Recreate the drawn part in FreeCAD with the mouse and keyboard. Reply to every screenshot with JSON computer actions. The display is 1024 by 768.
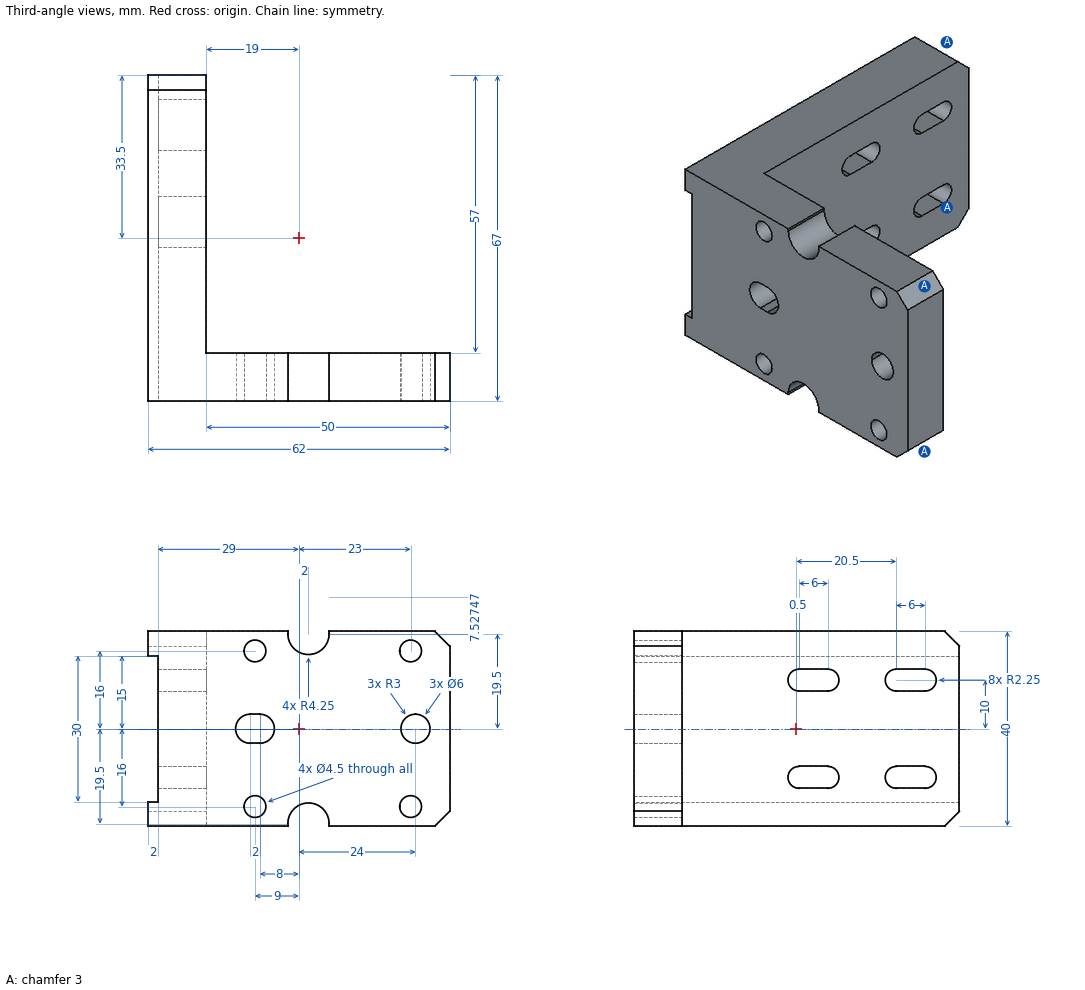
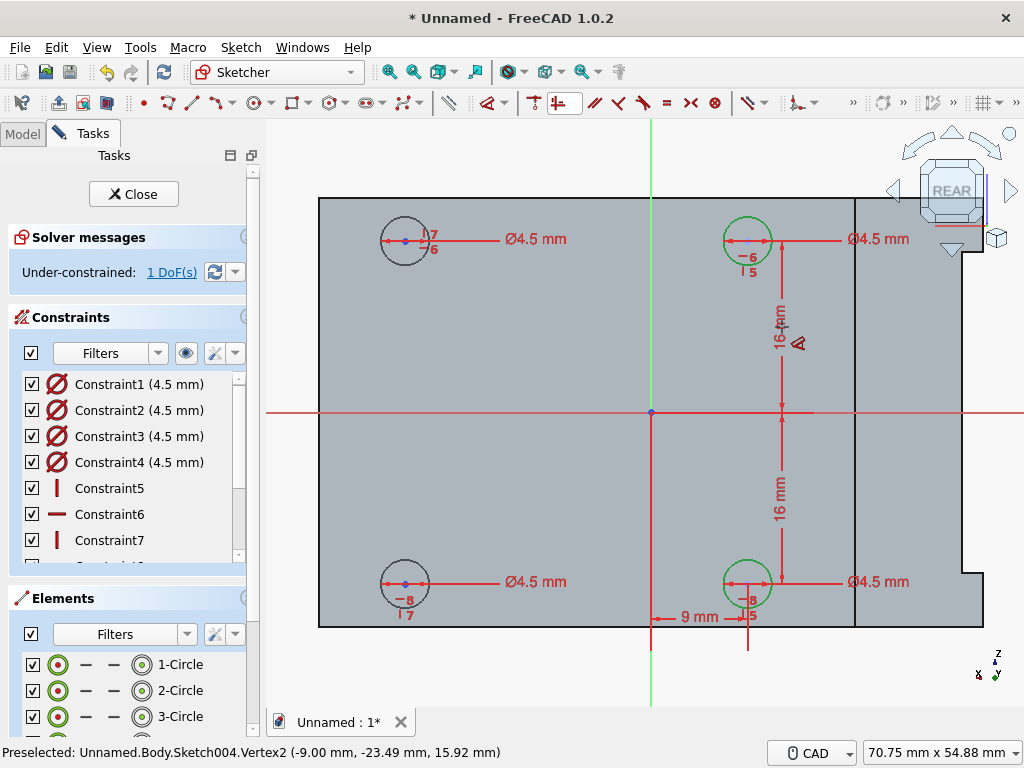
{"action": "left_click", "coordinate": [405, 241]}
{"action": "left_click", "coordinate": [528, 207]}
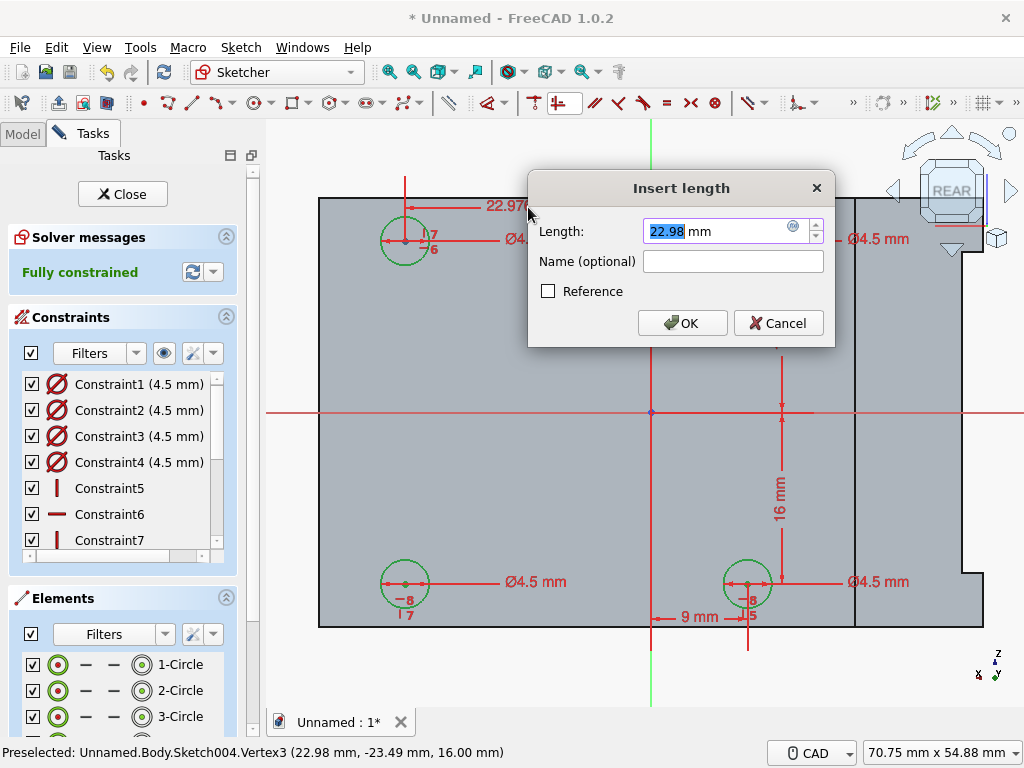
{"action": "type", "text": "23"}
{"action": "key", "text": "Return"}
{"action": "key", "text": "Escape"}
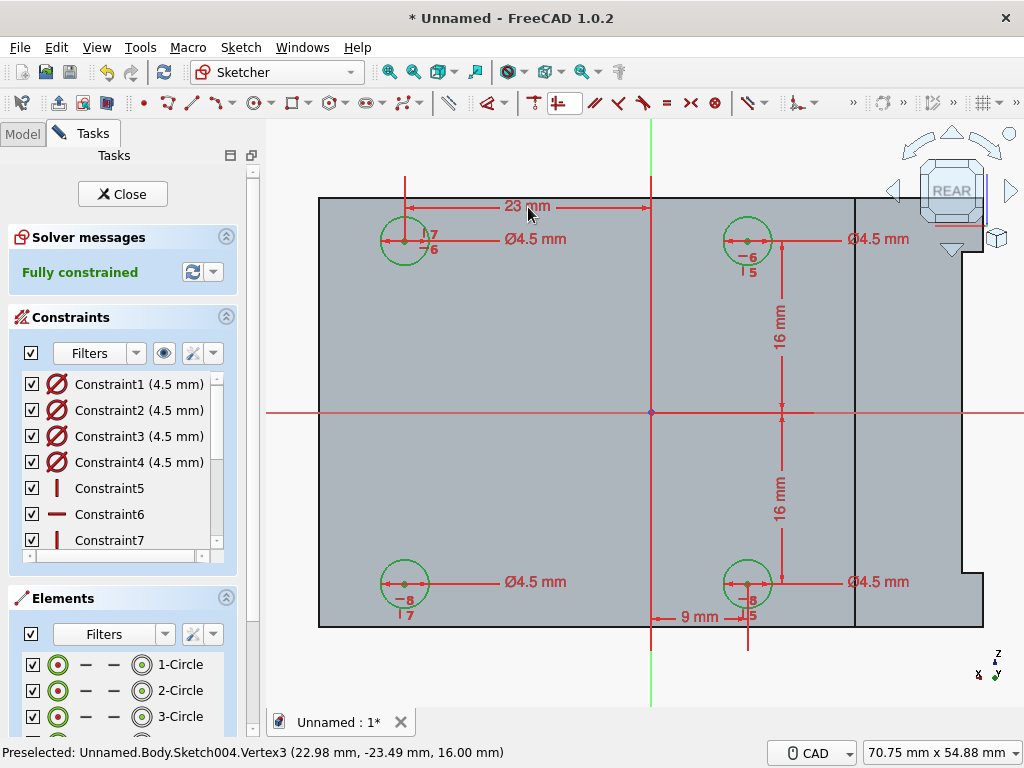
{"action": "left_click", "coordinate": [123, 194]}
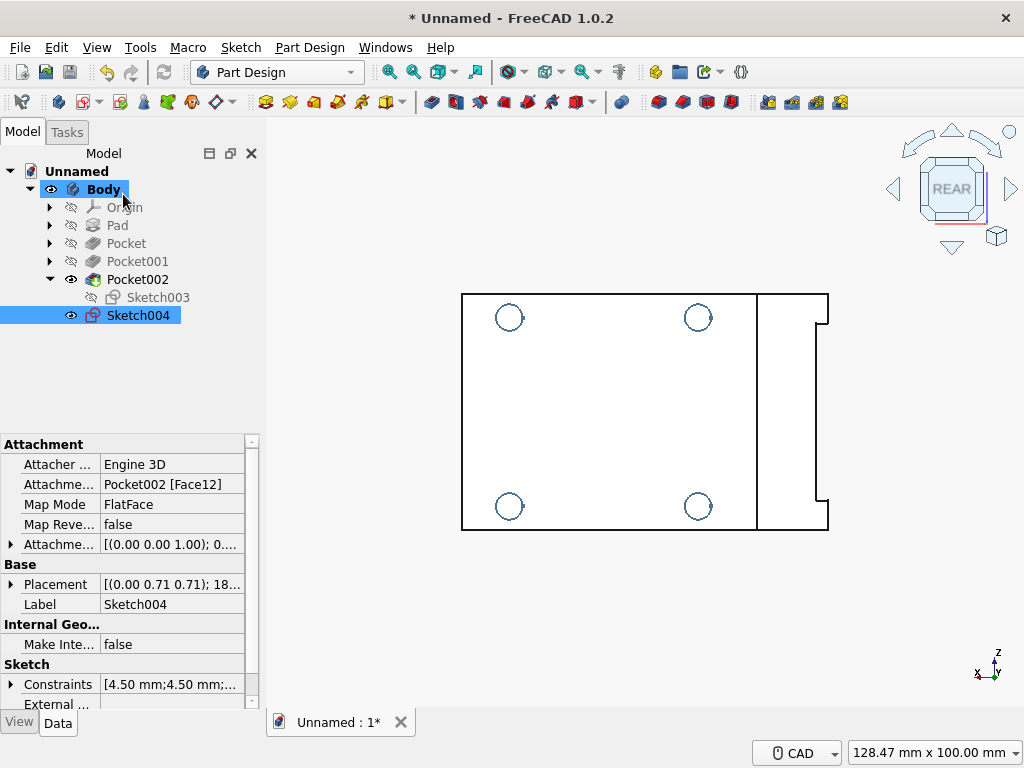
{"action": "left_click", "coordinate": [456, 102]}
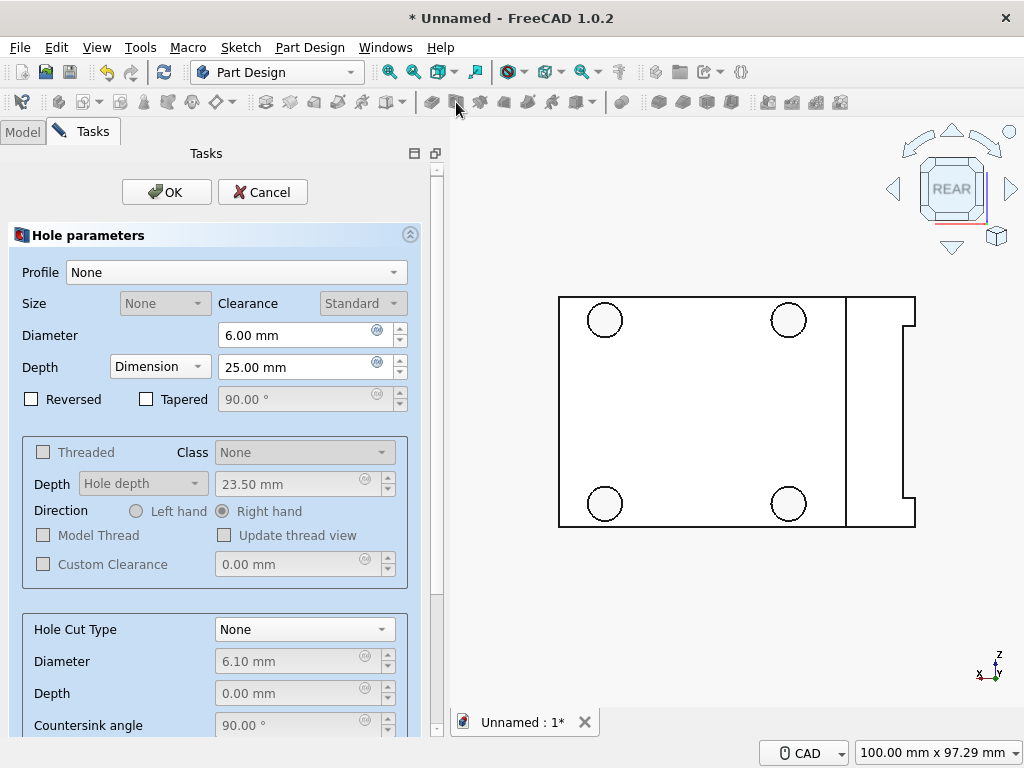
{"action": "triple_click", "coordinate": [305, 335]}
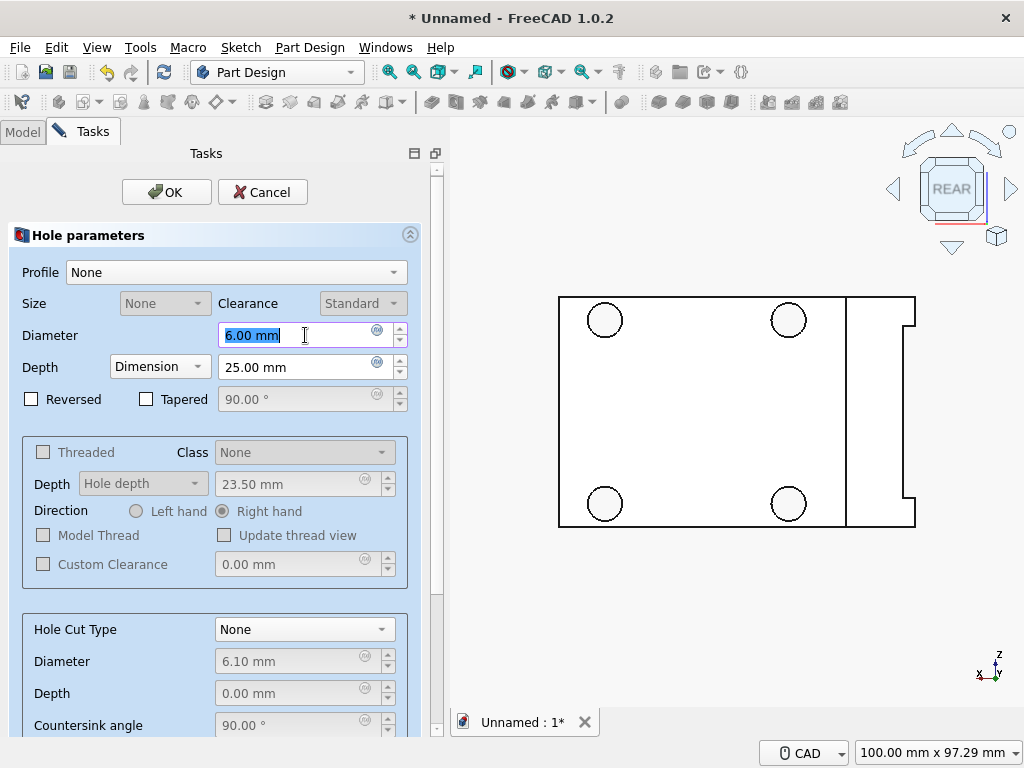
{"action": "type", "text": "4.5"}
{"action": "key", "text": "Tab"}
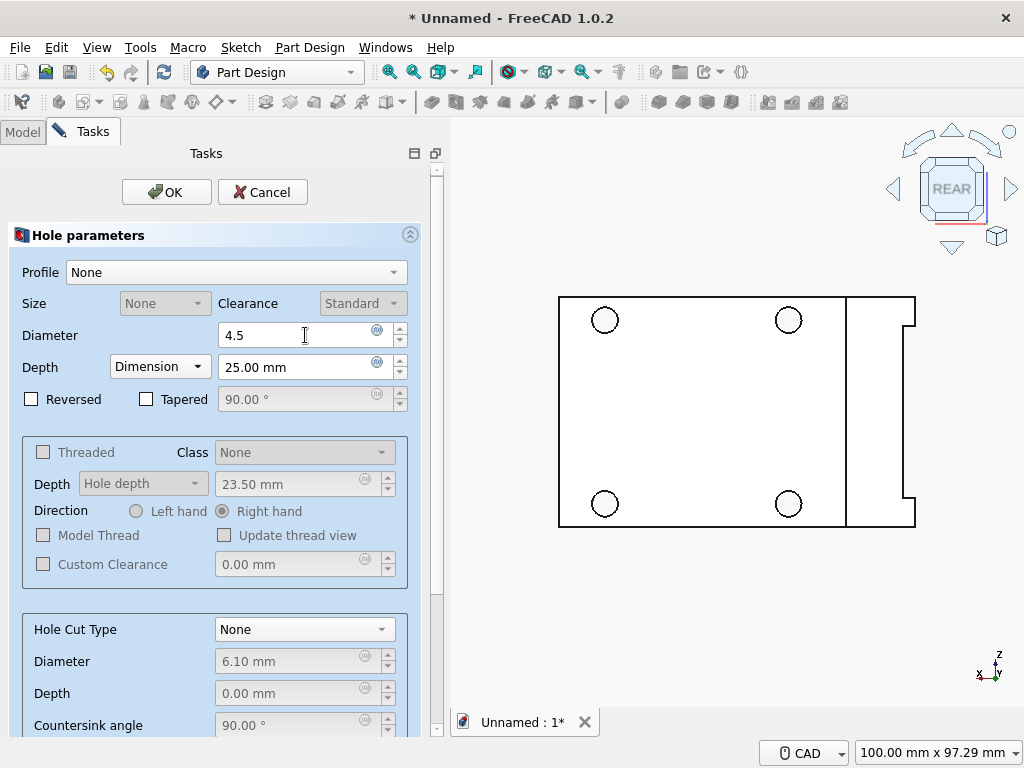
{"action": "left_click", "coordinate": [161, 366]}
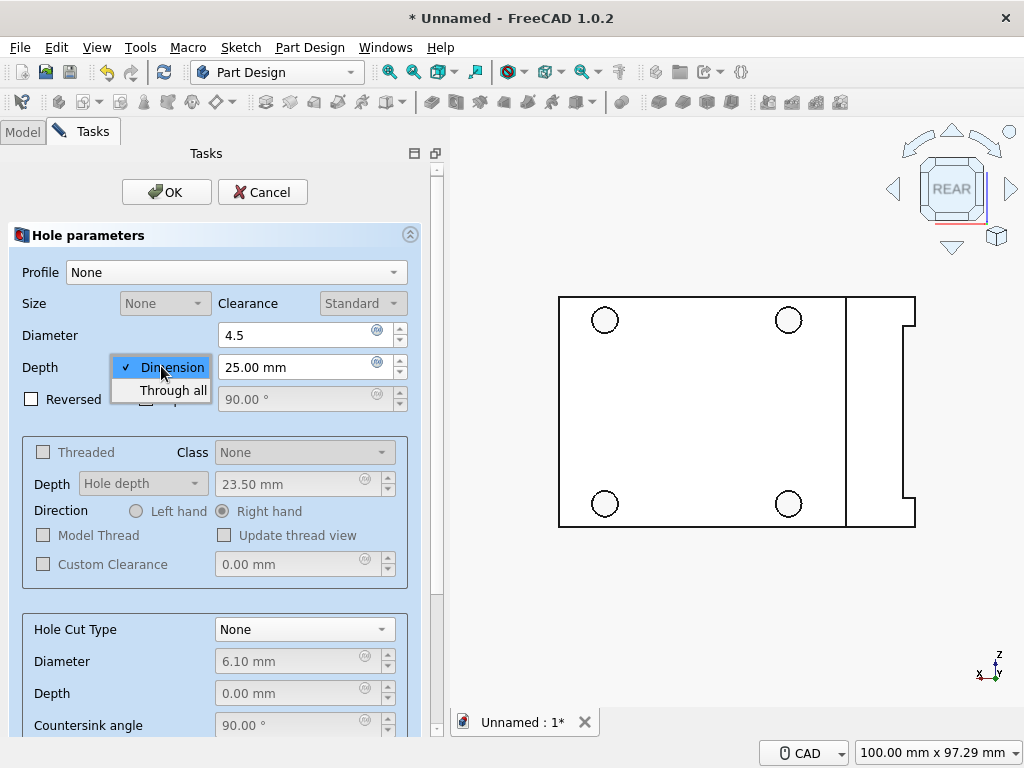
{"action": "left_click", "coordinate": [160, 390]}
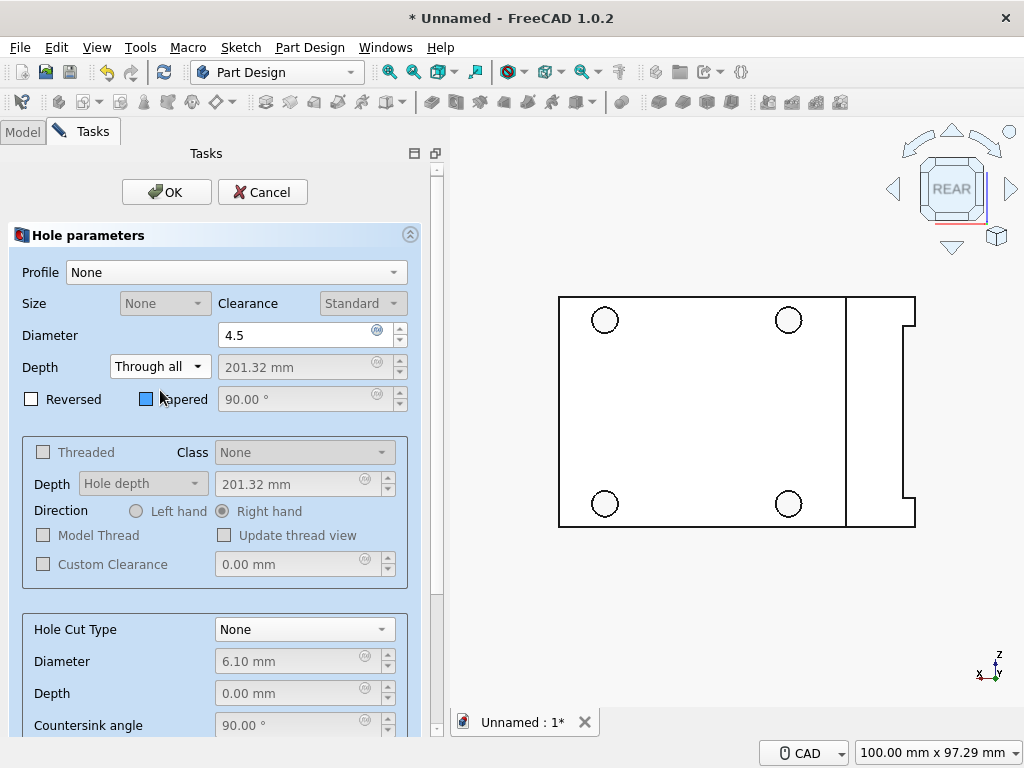
{"action": "left_click", "coordinate": [167, 192]}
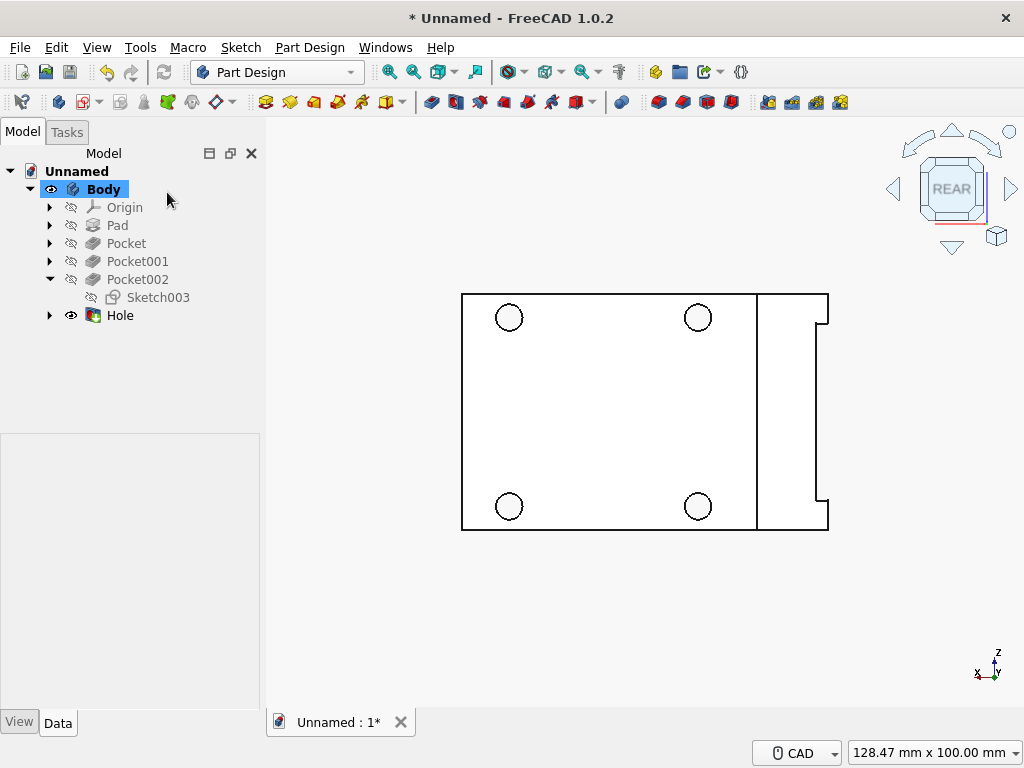
{"action": "left_click", "coordinate": [610, 411]}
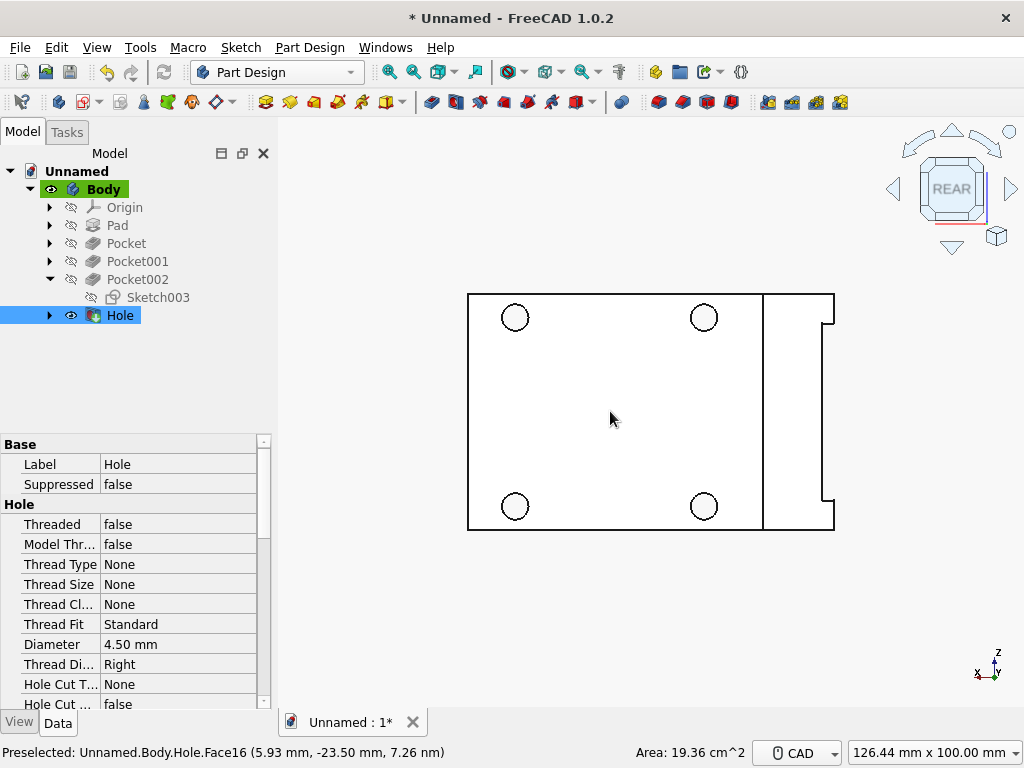
{"action": "left_click", "coordinate": [84, 102]}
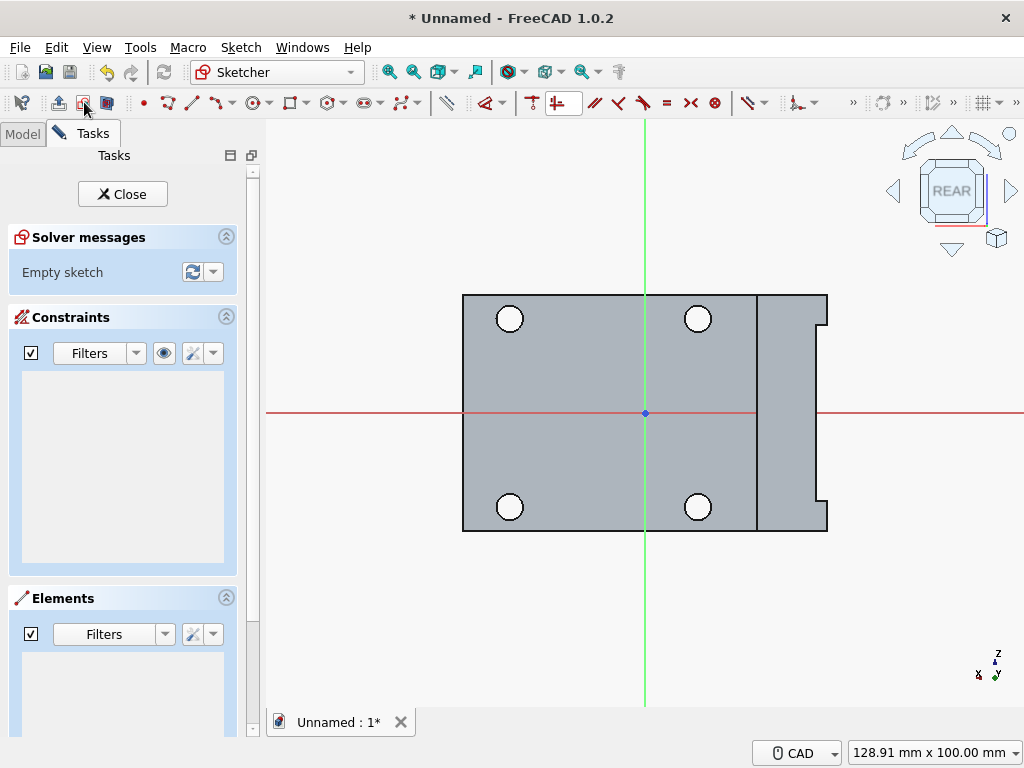
{"action": "scroll", "coordinate": [637, 413], "scroll_direction": "up", "scroll_amount": 3}